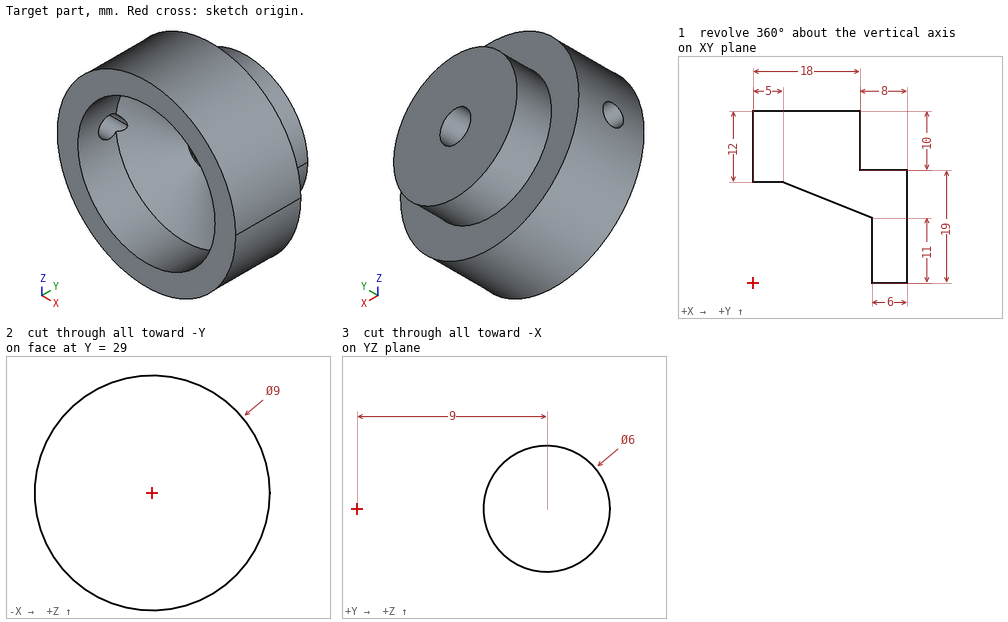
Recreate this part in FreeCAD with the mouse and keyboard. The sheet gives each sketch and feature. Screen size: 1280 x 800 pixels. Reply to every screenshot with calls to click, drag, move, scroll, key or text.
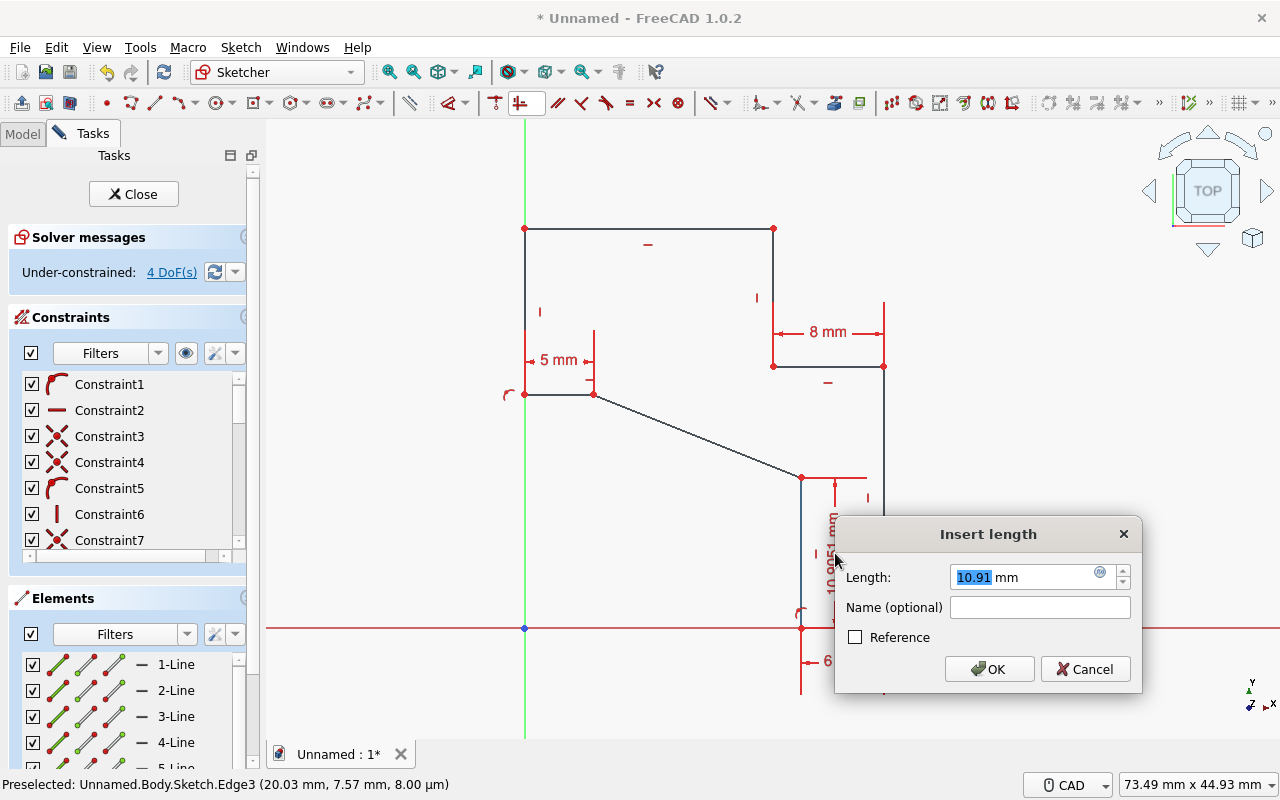
text(11)
key(Return)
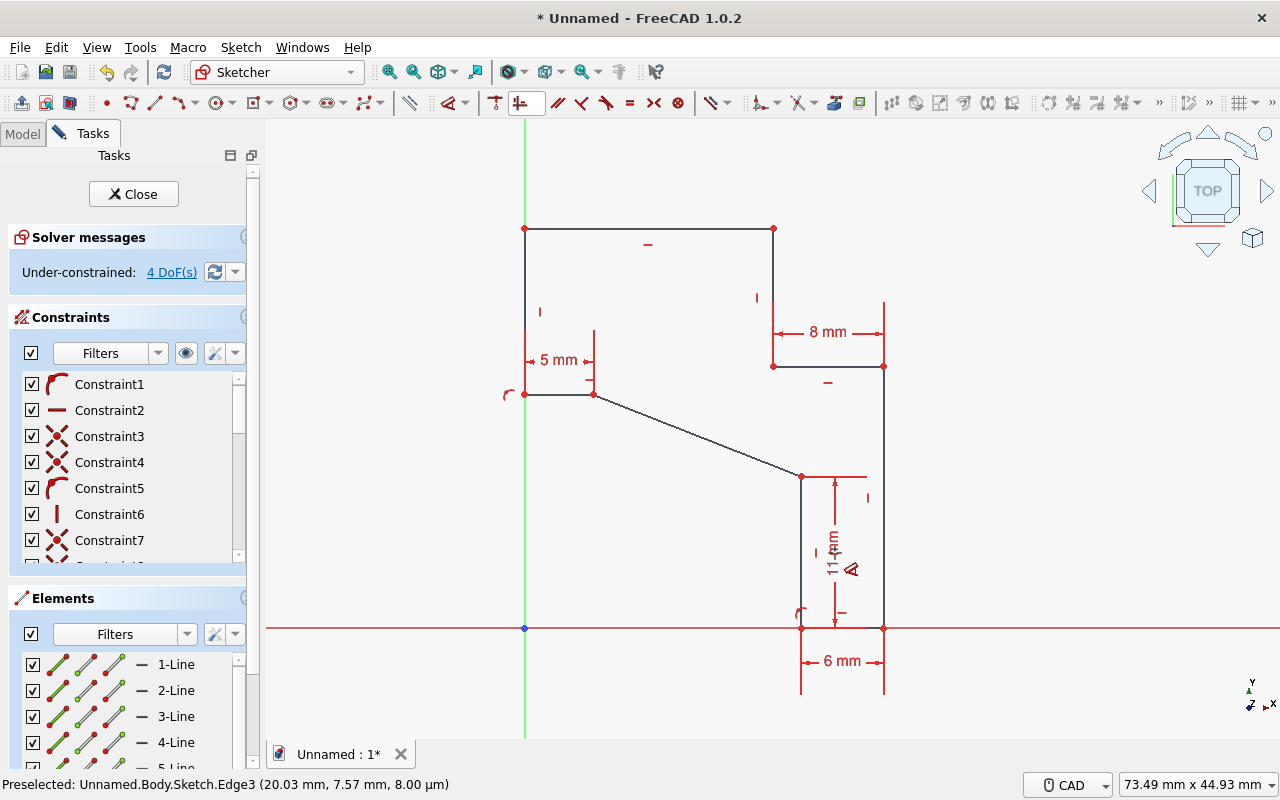
click(884, 550)
click(918, 498)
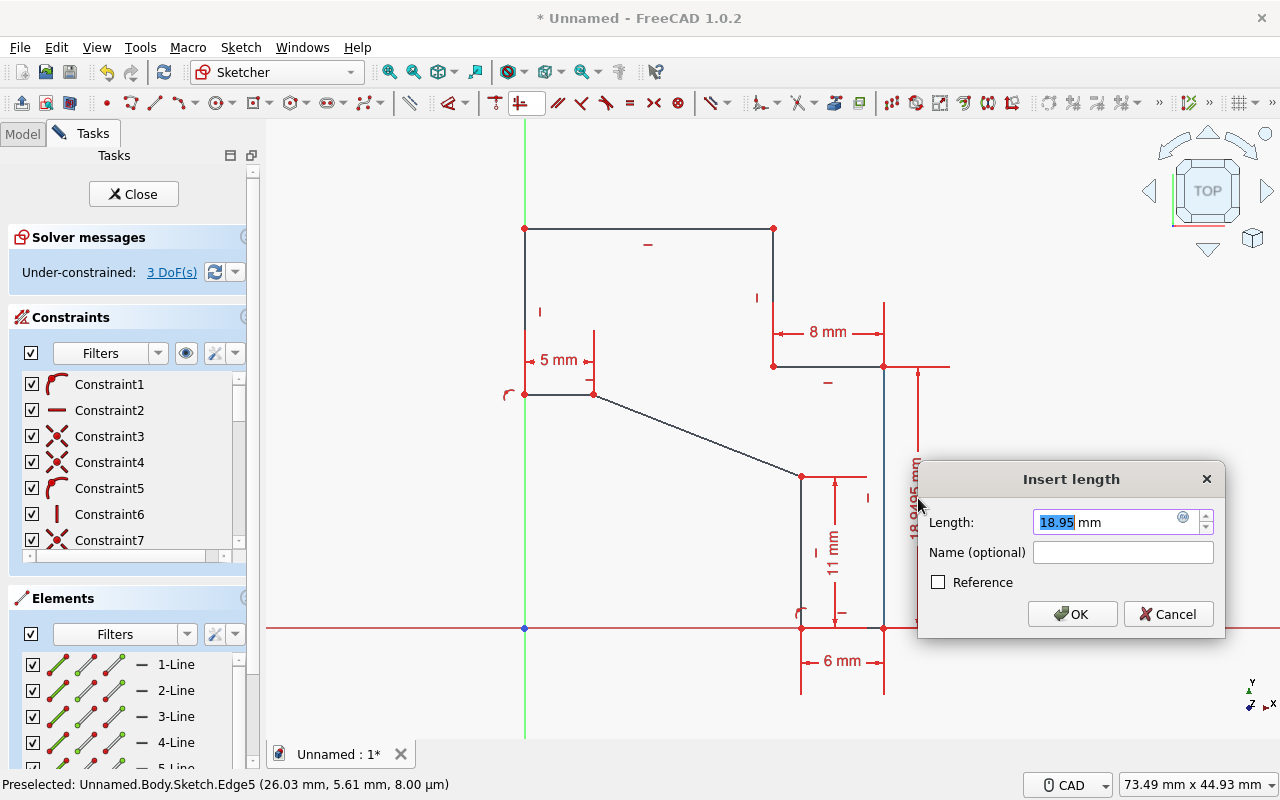
text(19)
key(Return)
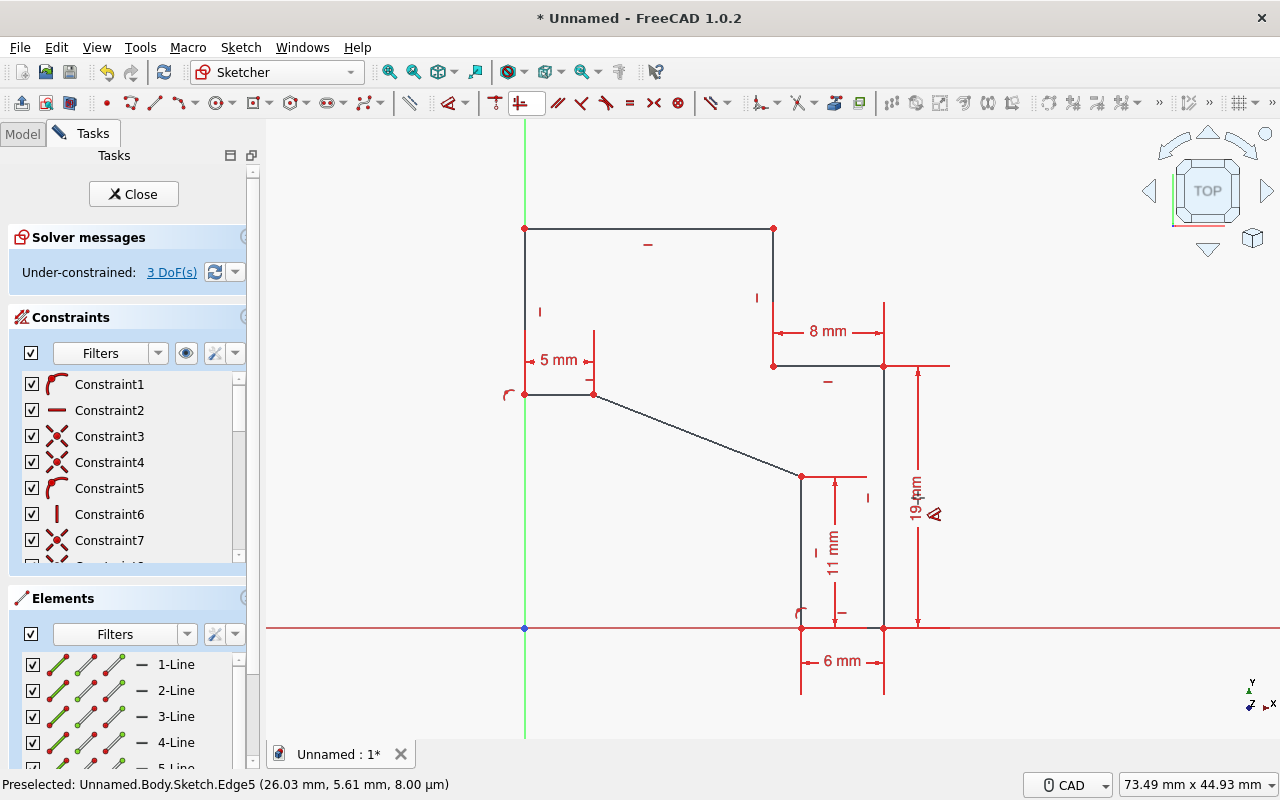
click(773, 325)
click(807, 298)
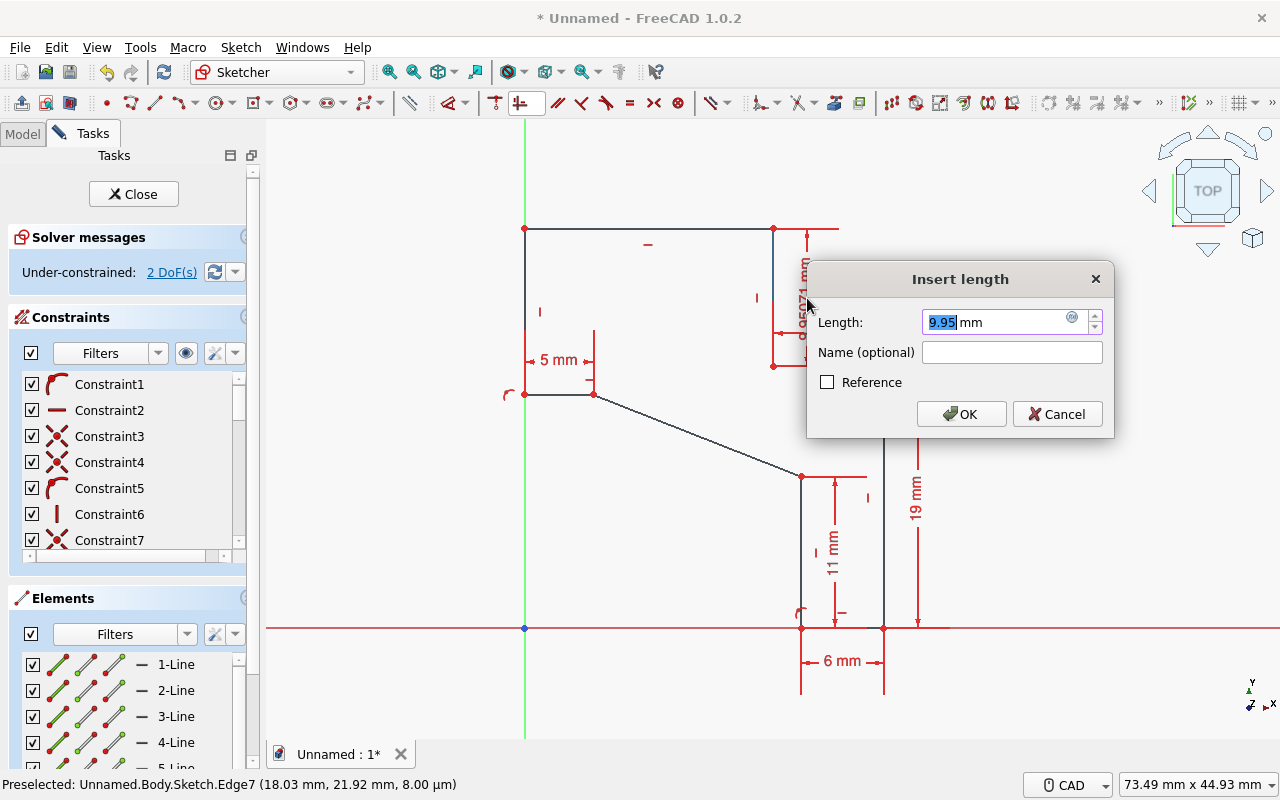
text(10)
key(Return)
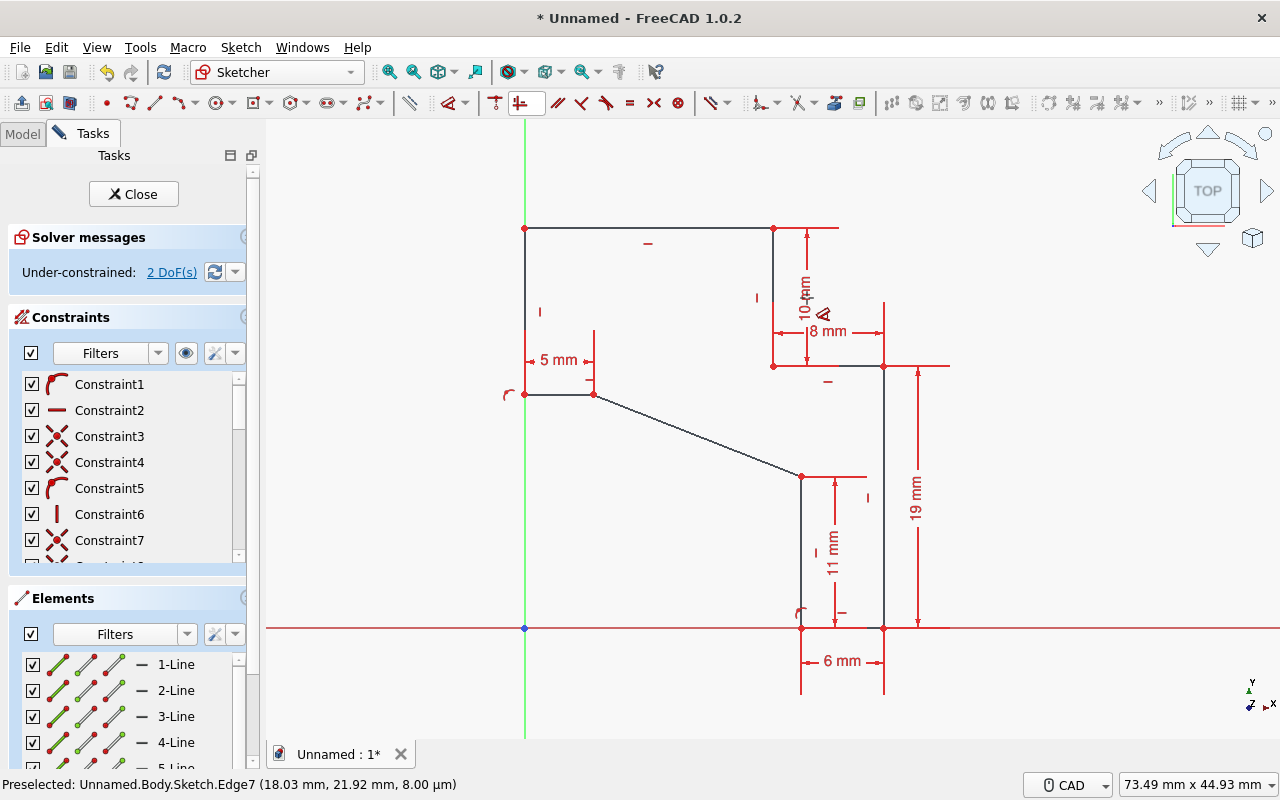
click(699, 228)
click(649, 194)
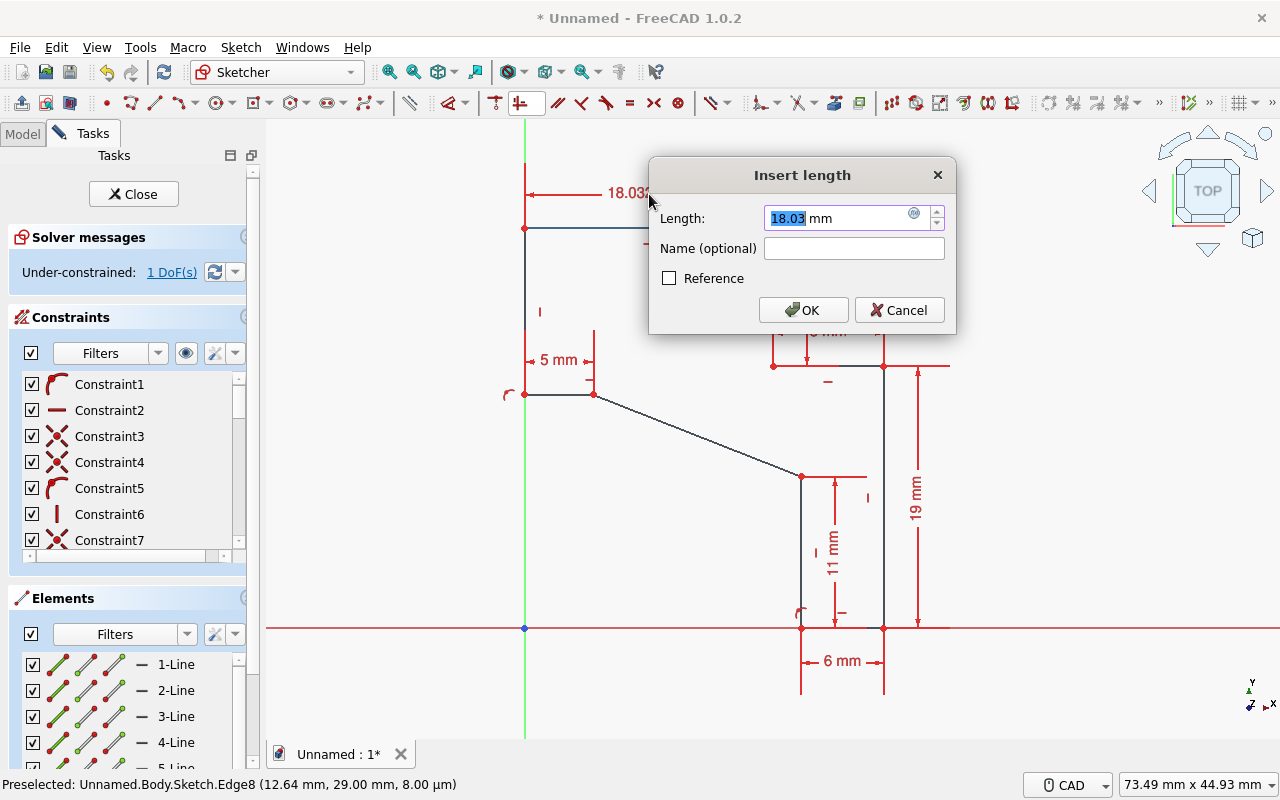
text(18)
key(Return)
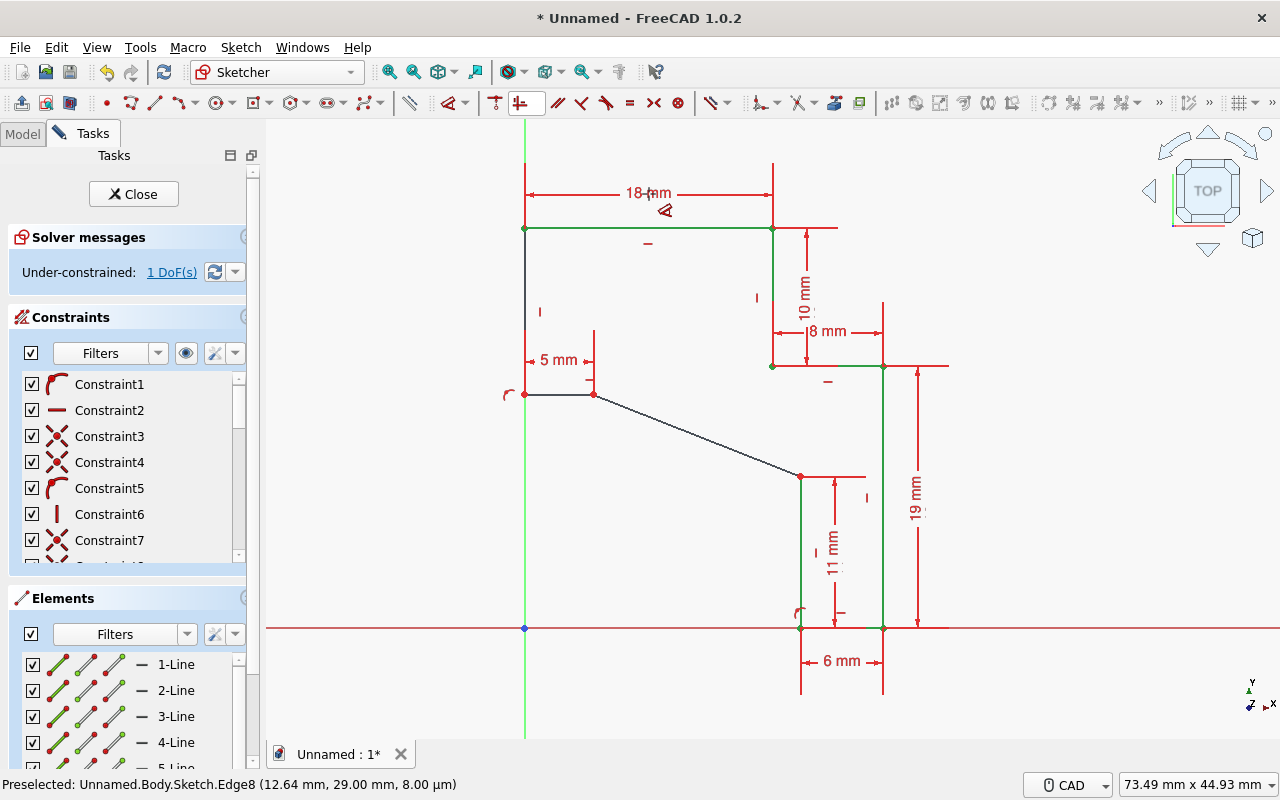
click(525, 278)
click(491, 312)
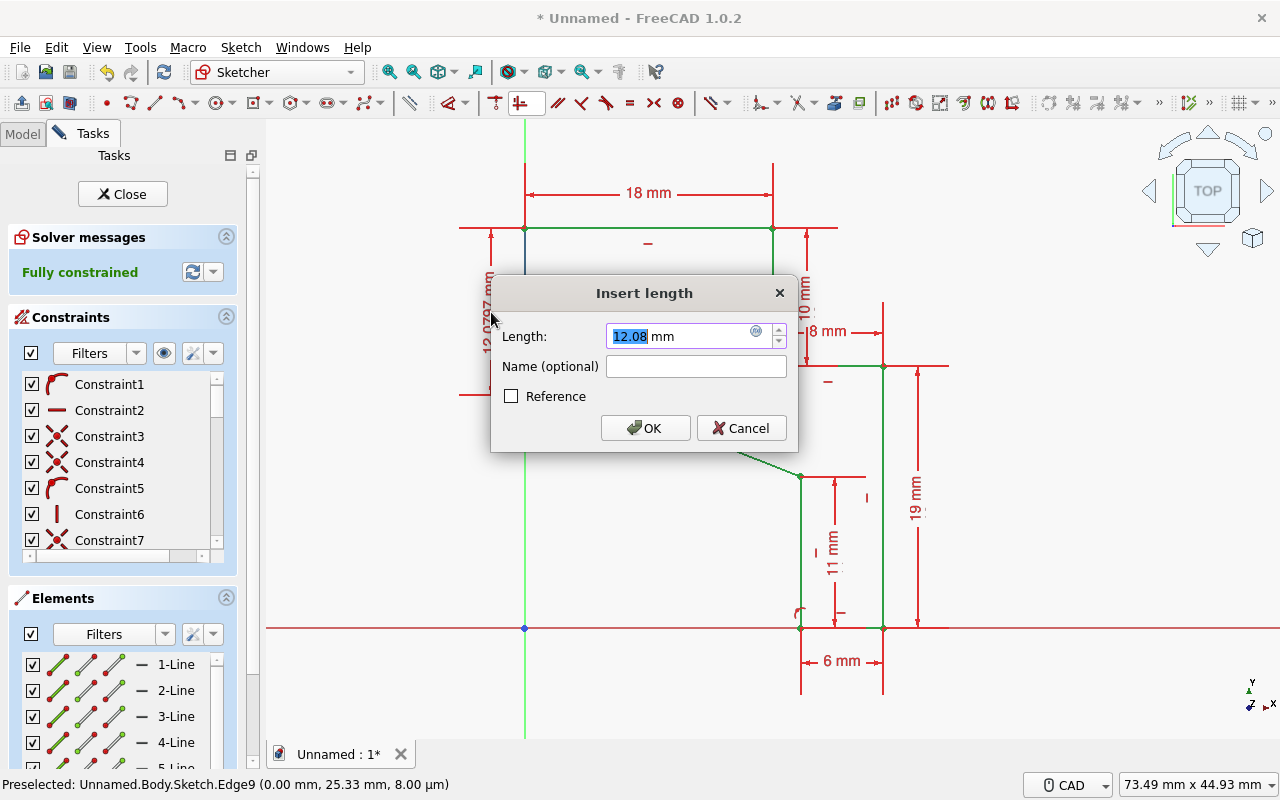
text(12)
key(Return)
key(Escape)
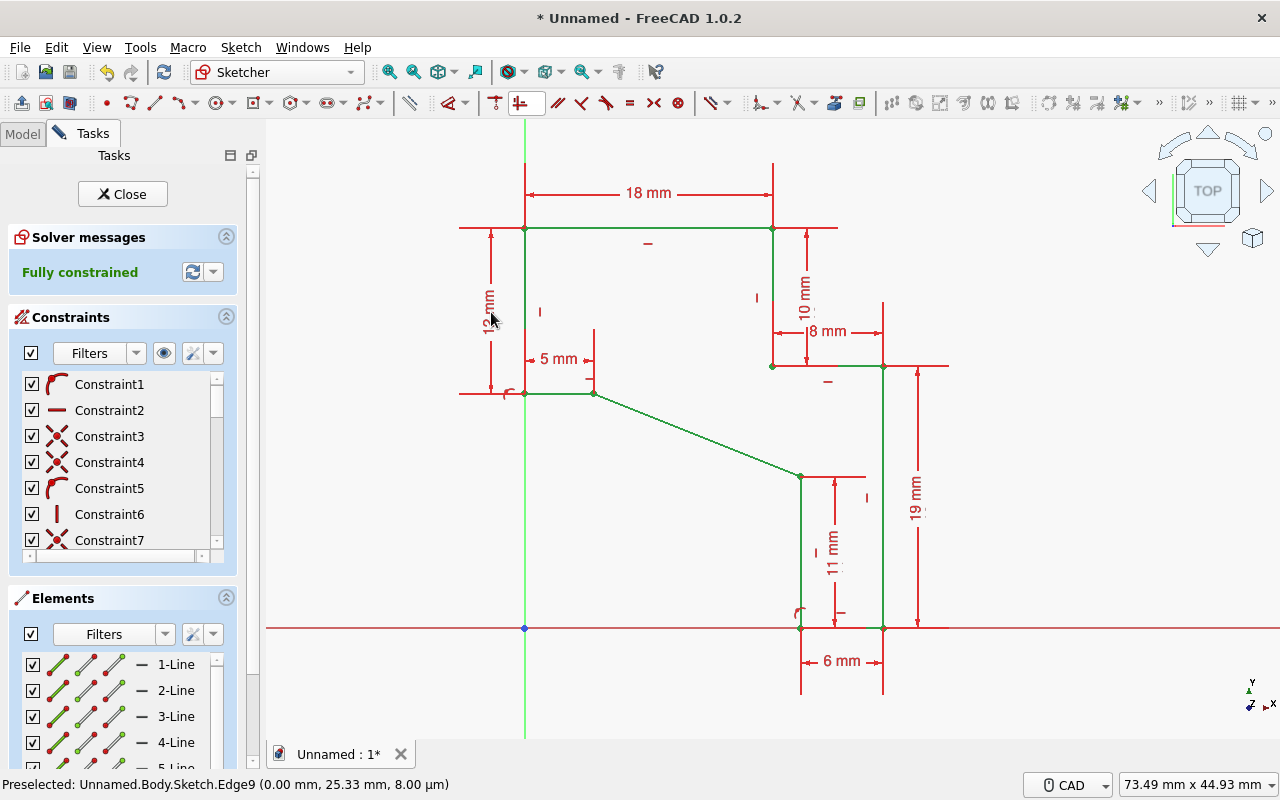
click(123, 194)